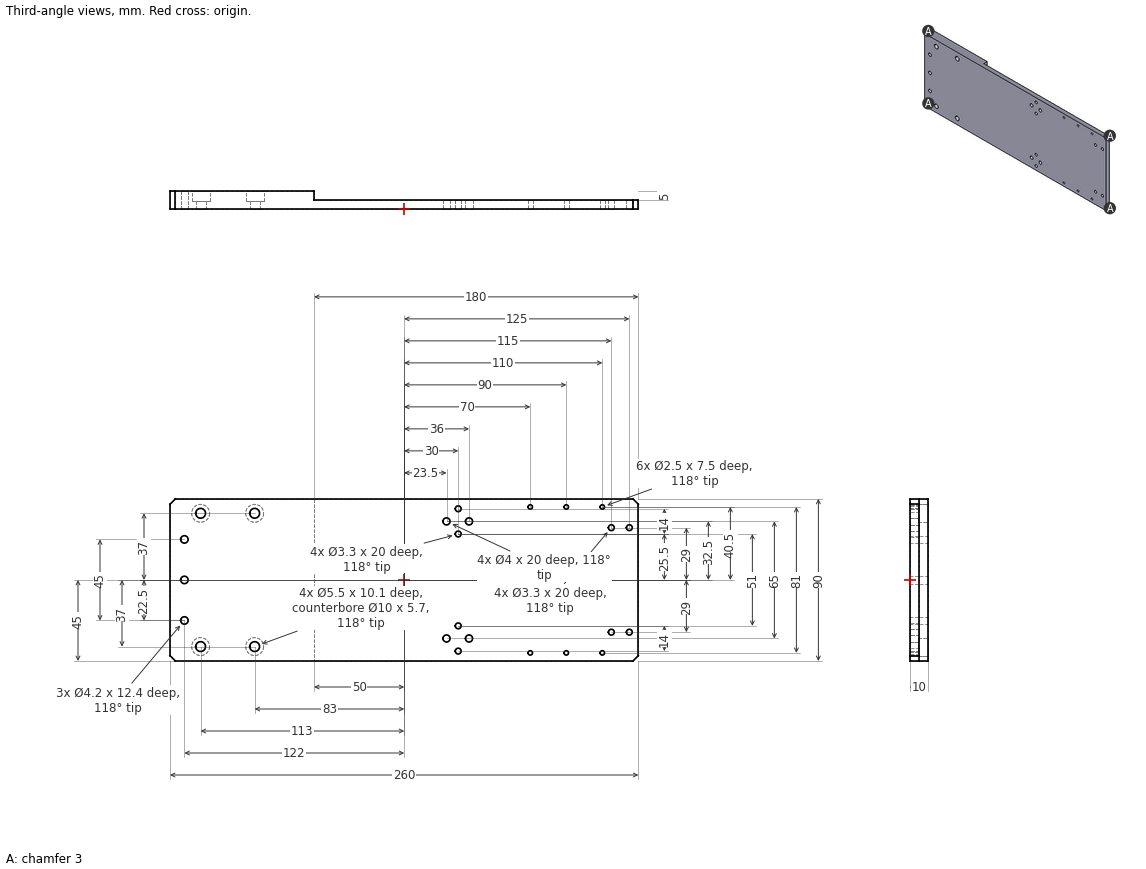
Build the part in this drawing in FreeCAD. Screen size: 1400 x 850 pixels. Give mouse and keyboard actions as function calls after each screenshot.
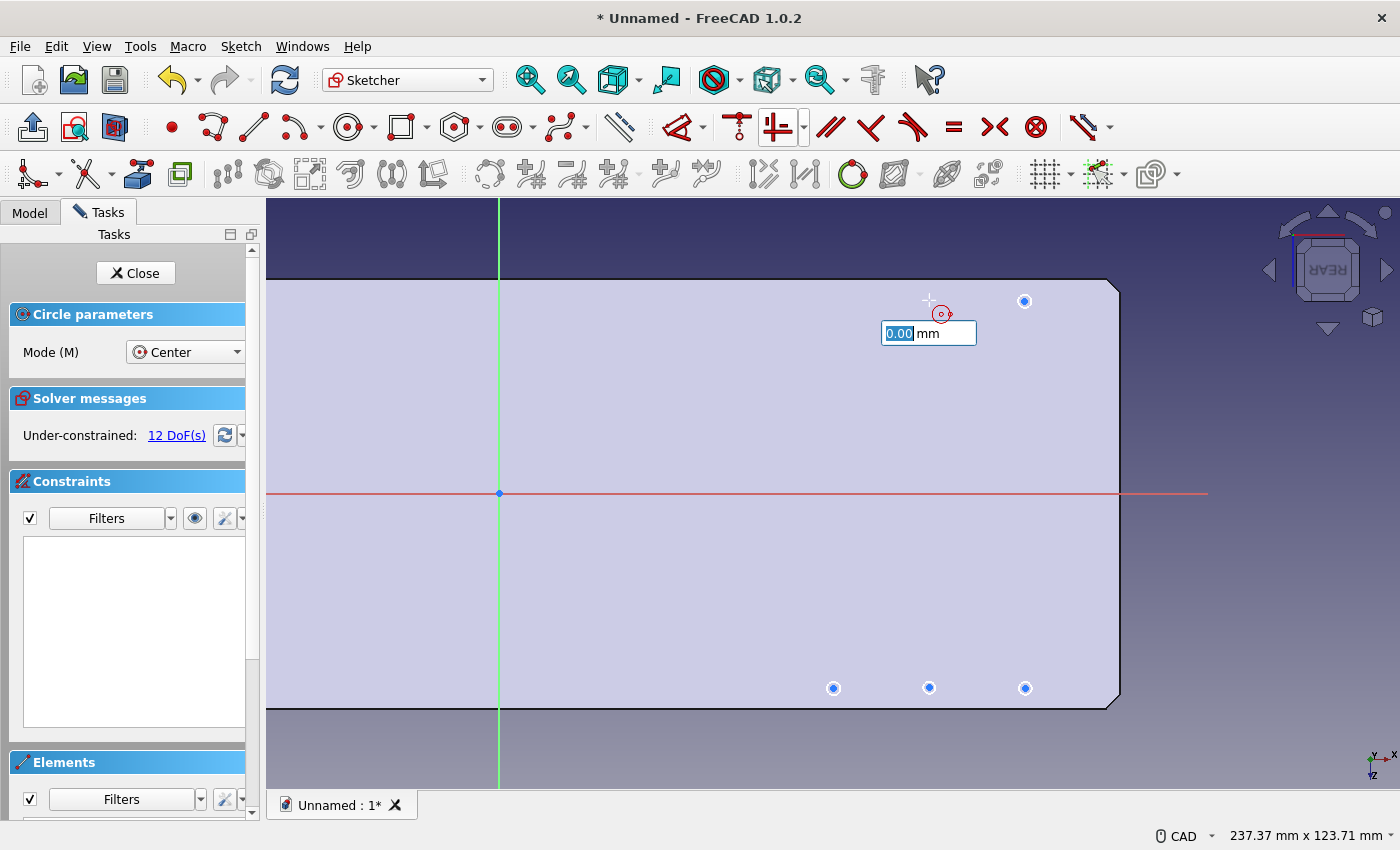
scroll(934, 296, up, 5)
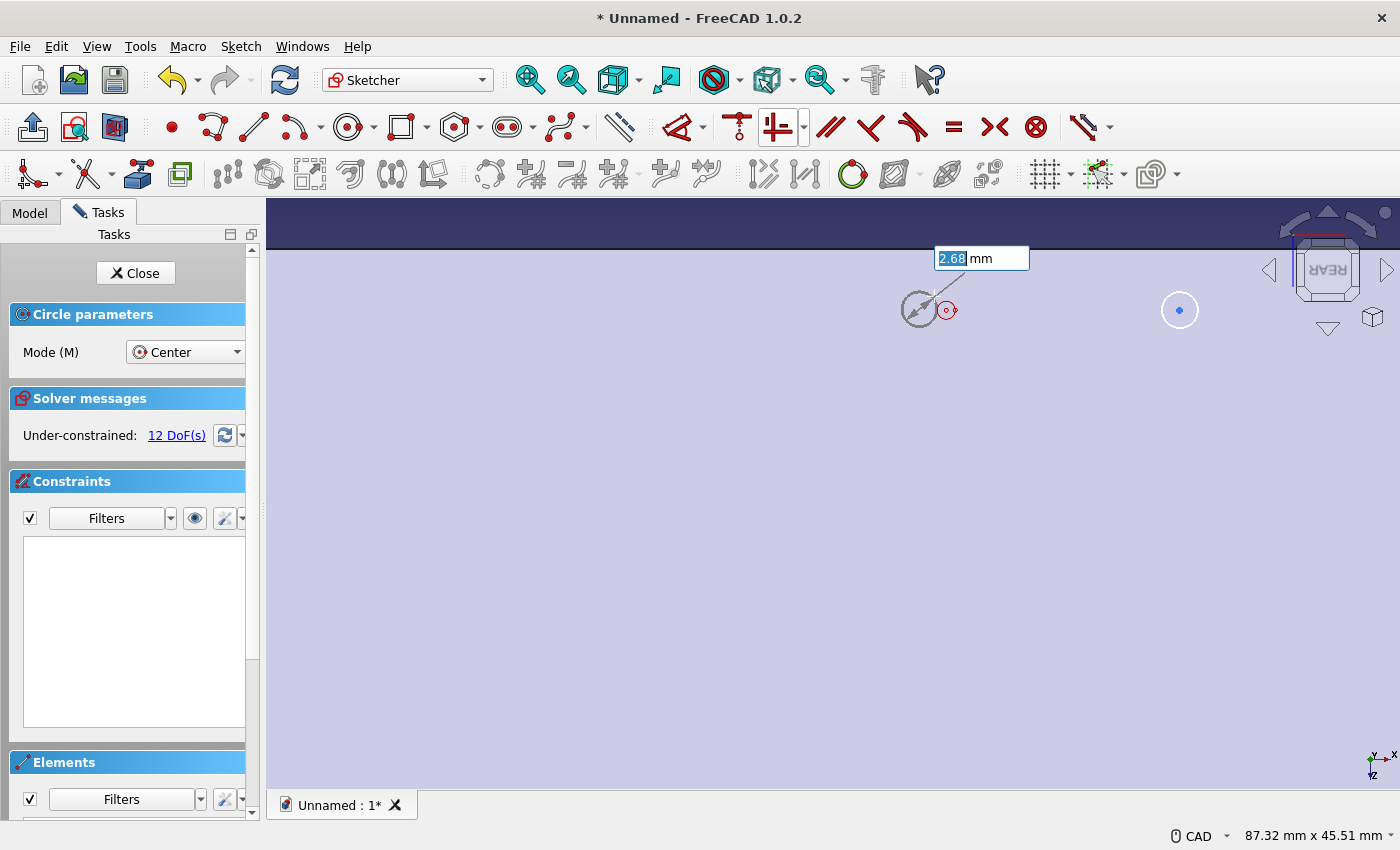
click(932, 296)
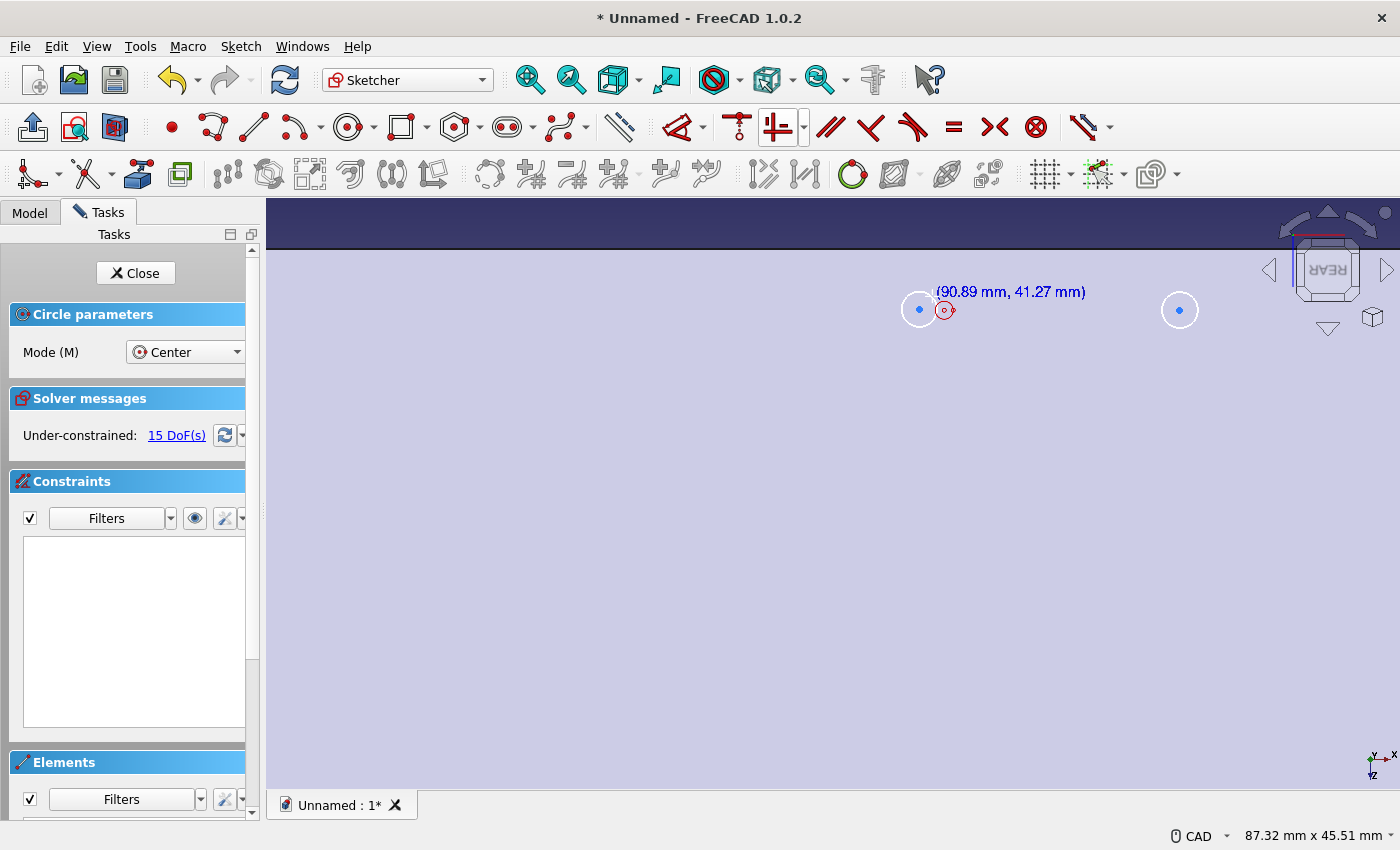
scroll(661, 307, up, 2)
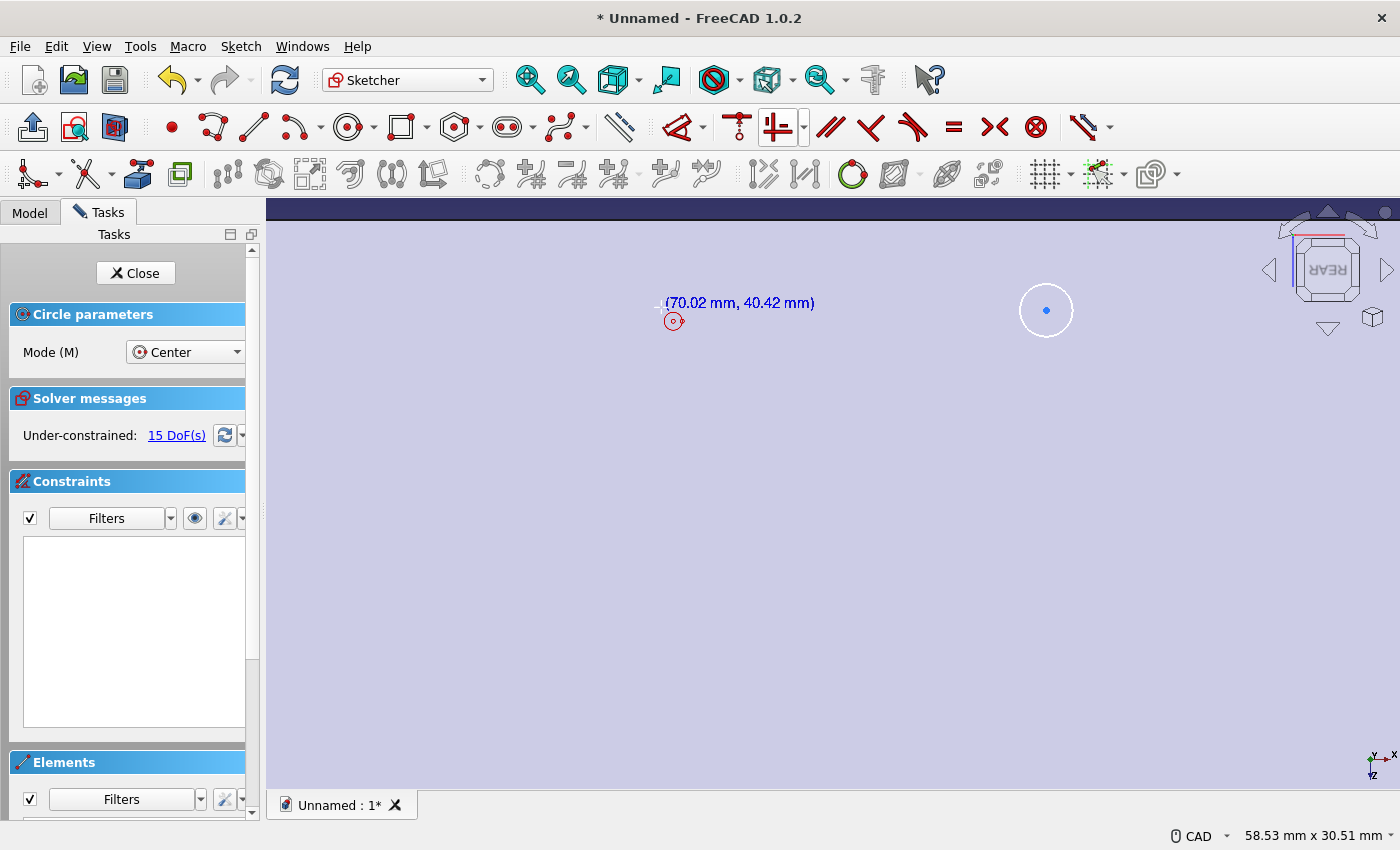
scroll(890, 298, down, 7)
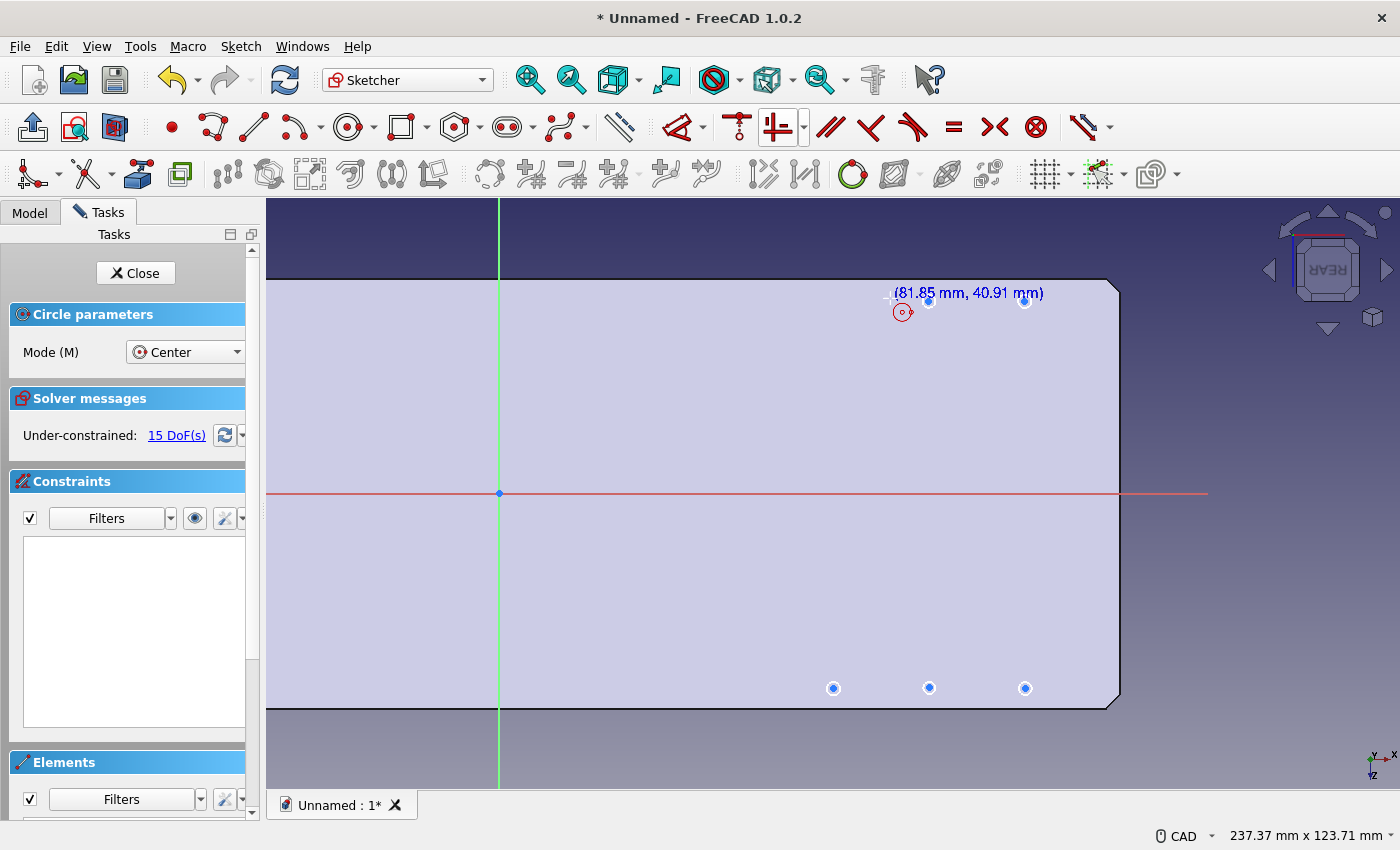
click(834, 300)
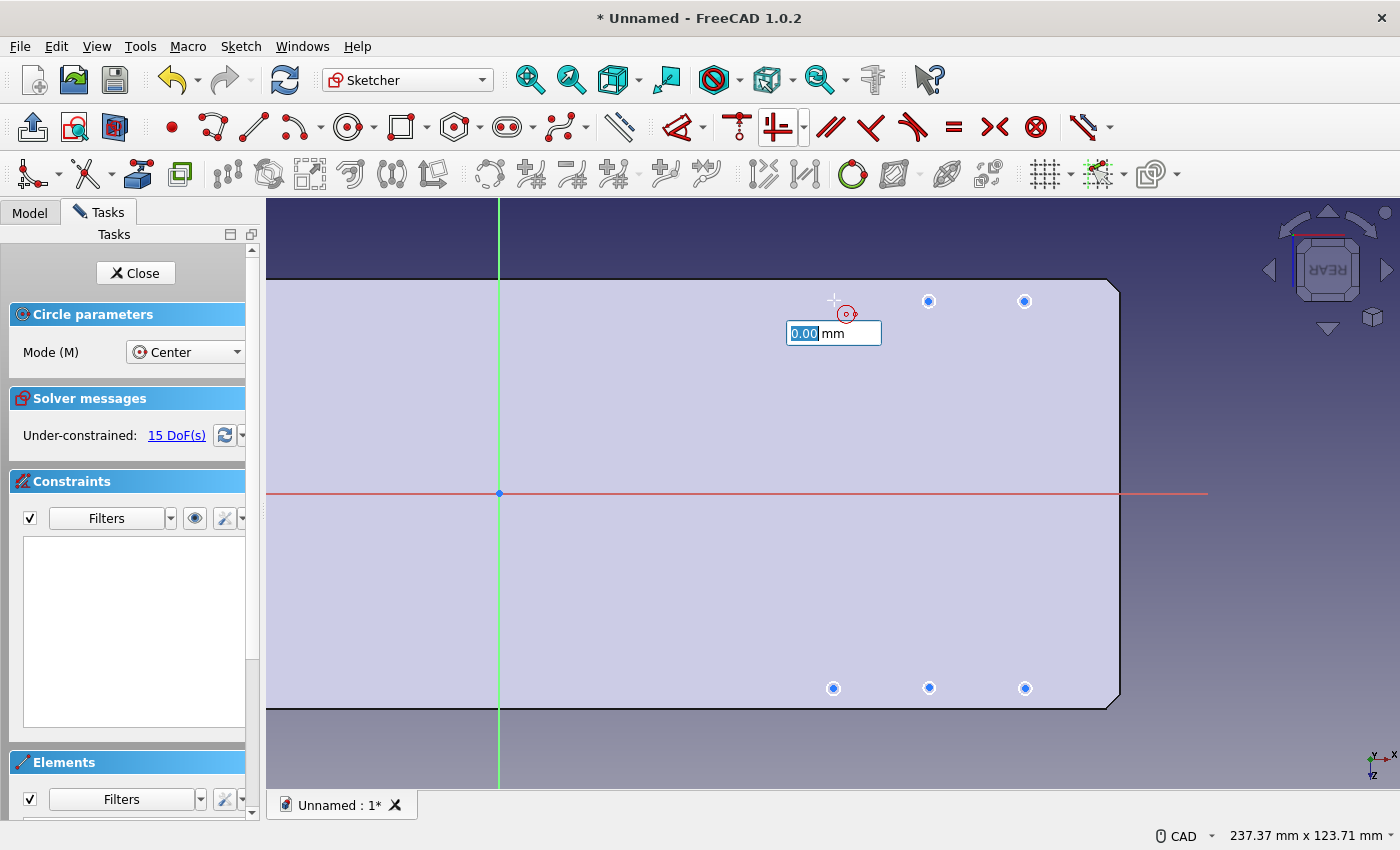
scroll(838, 296, up, 5)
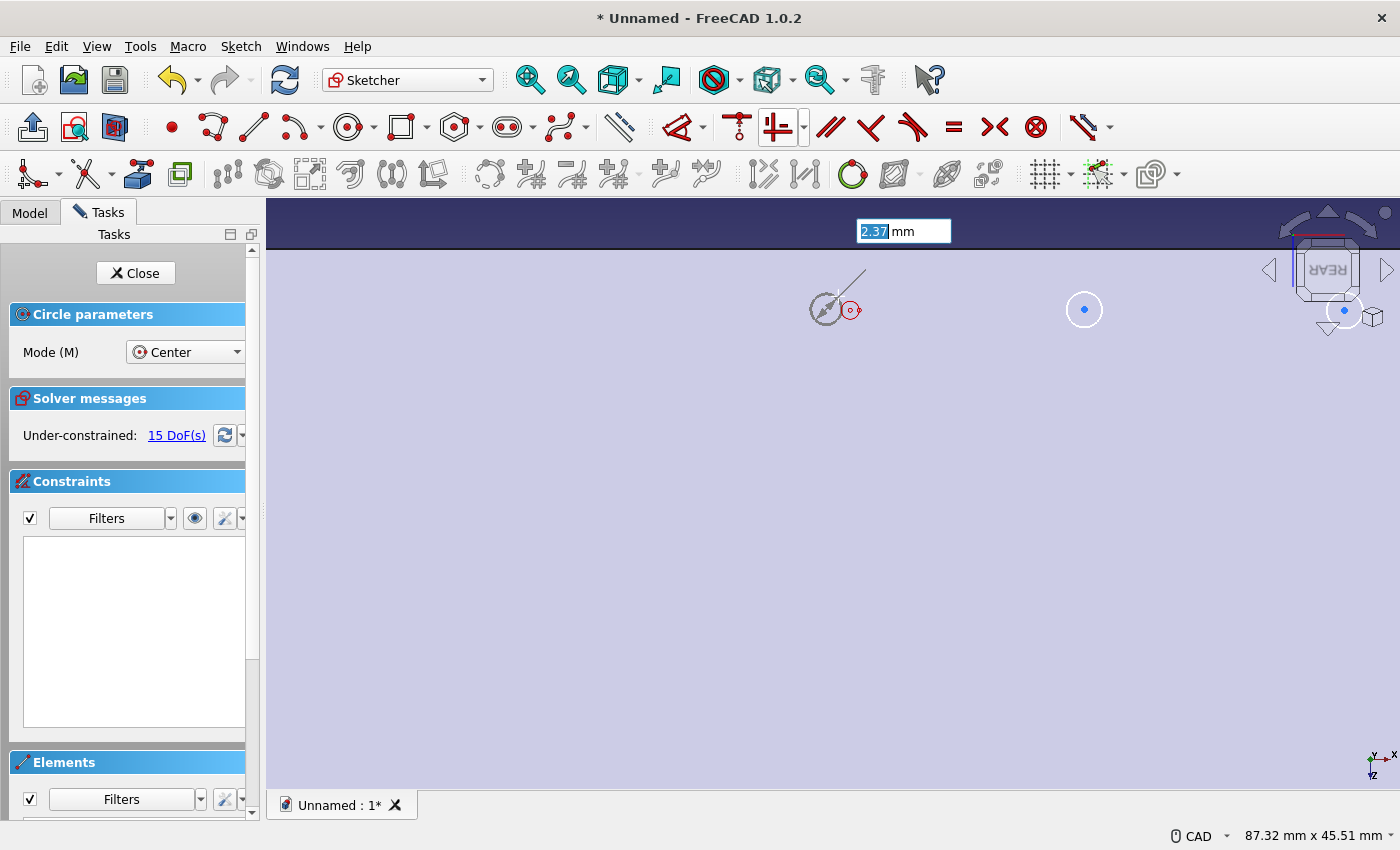
click(837, 296)
key(Escape)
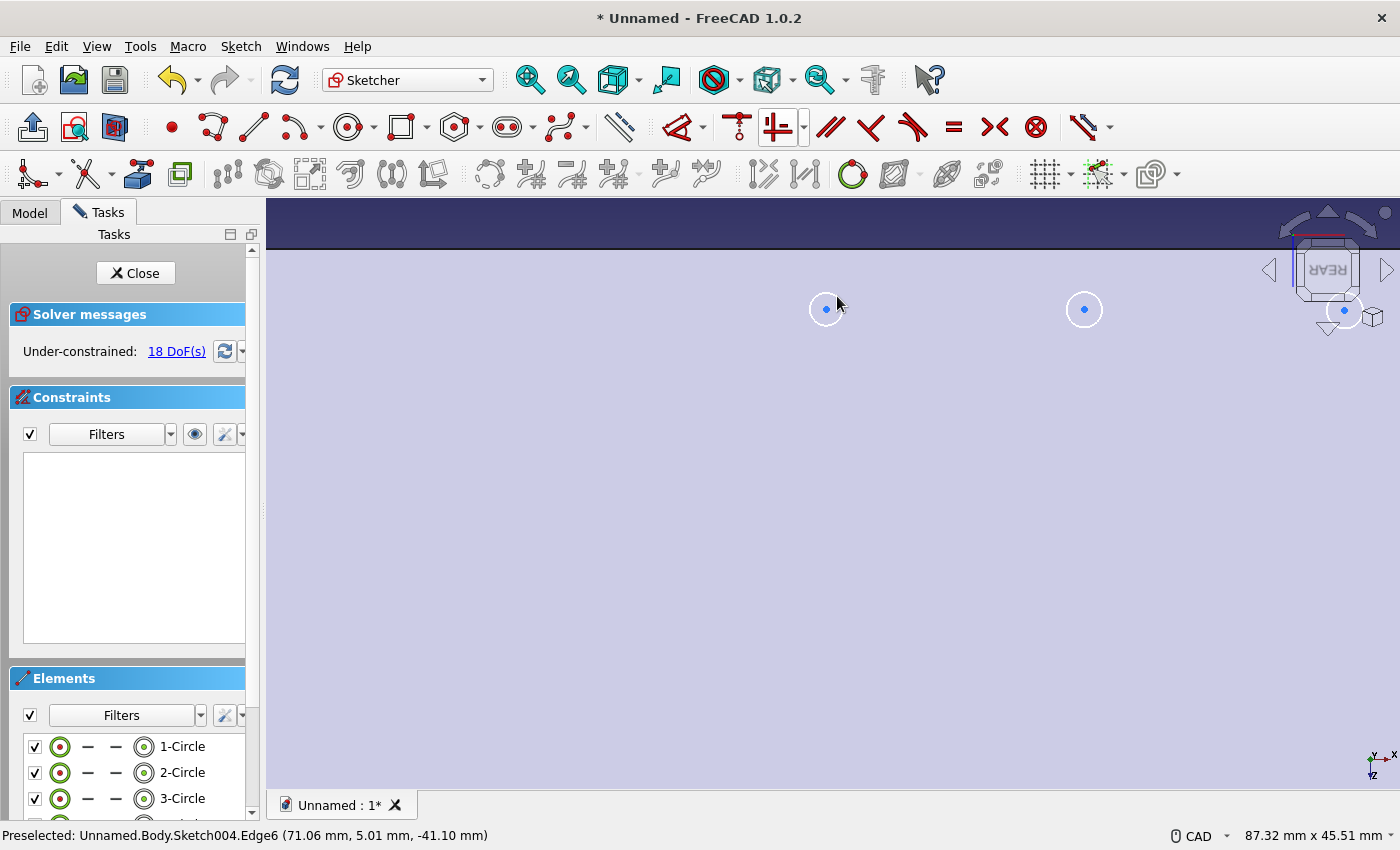
scroll(838, 296, down, 5)